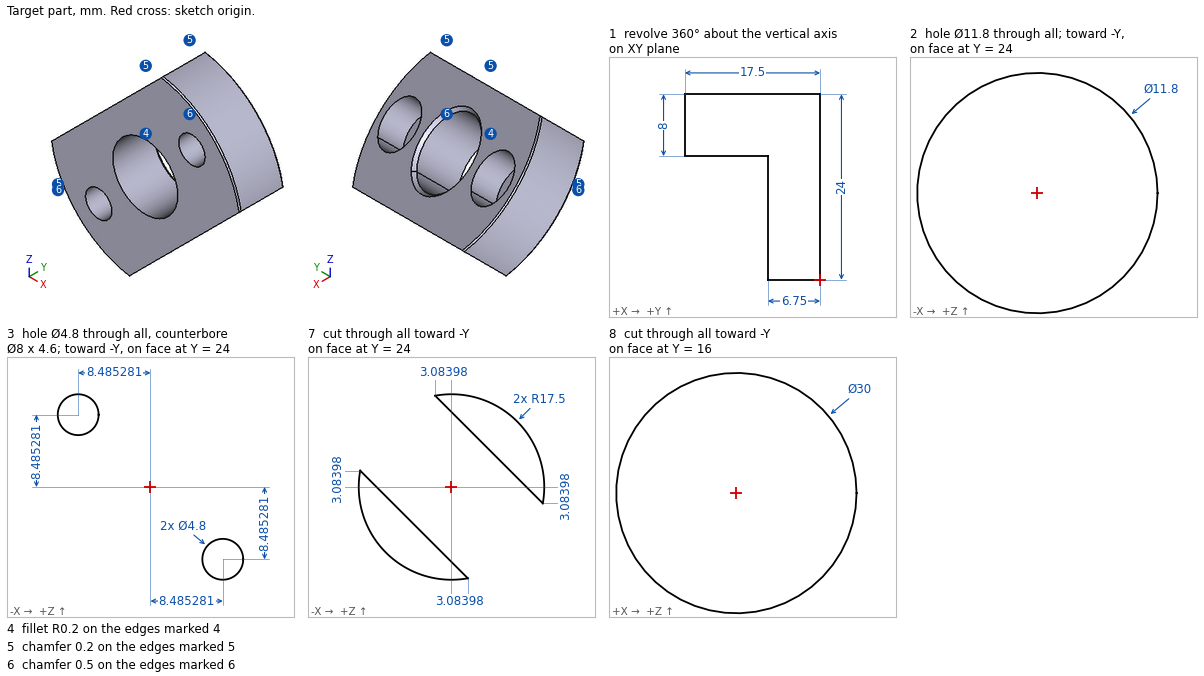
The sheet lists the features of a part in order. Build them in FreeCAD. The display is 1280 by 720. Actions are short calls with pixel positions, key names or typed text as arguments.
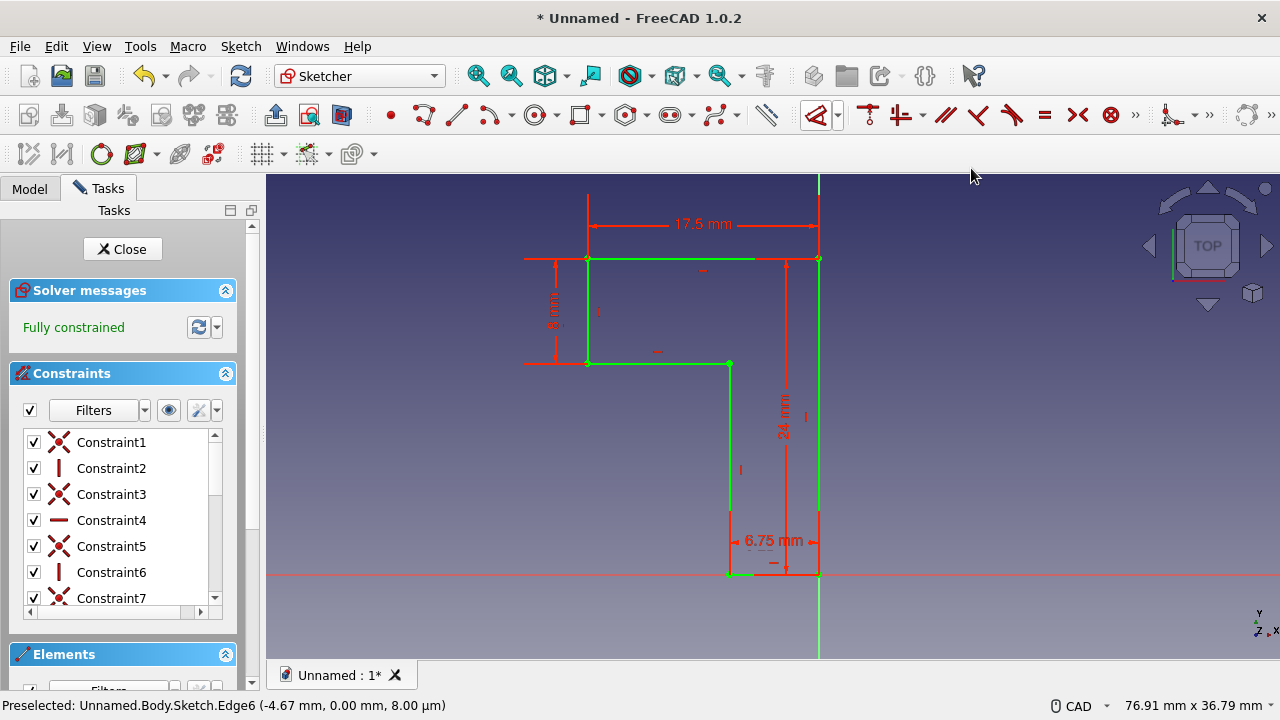
click(123, 249)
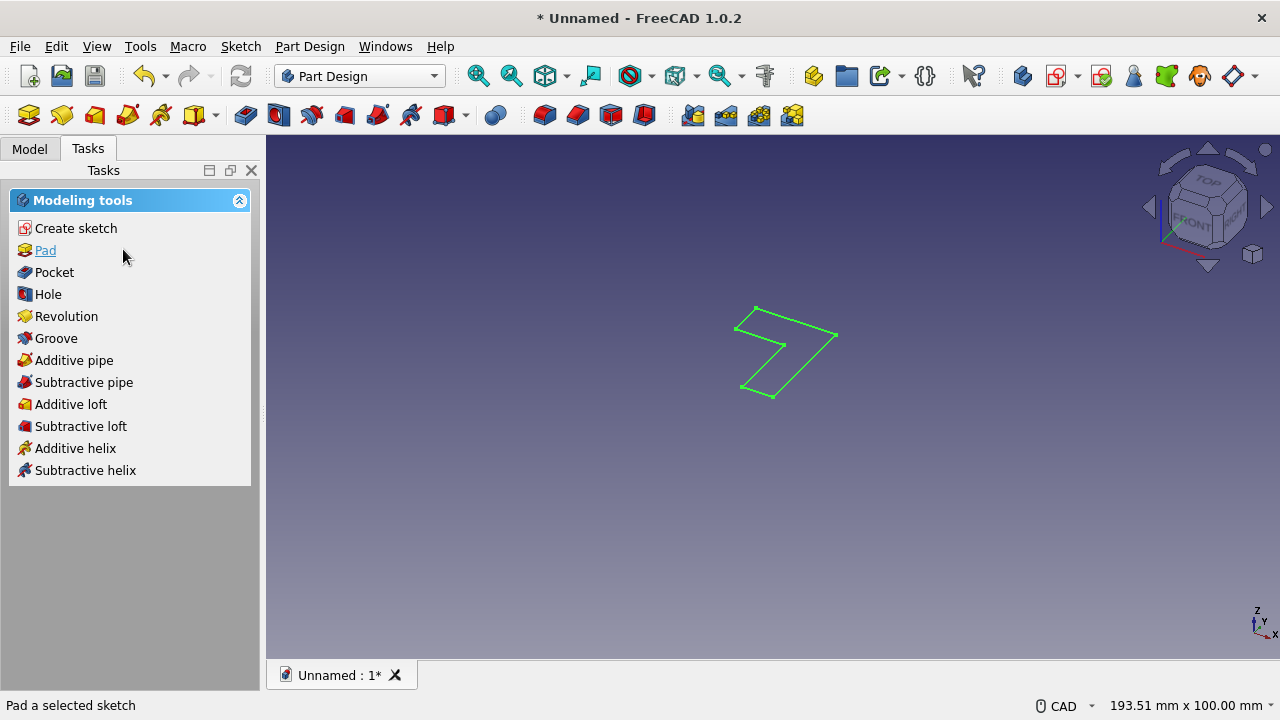
click(62, 116)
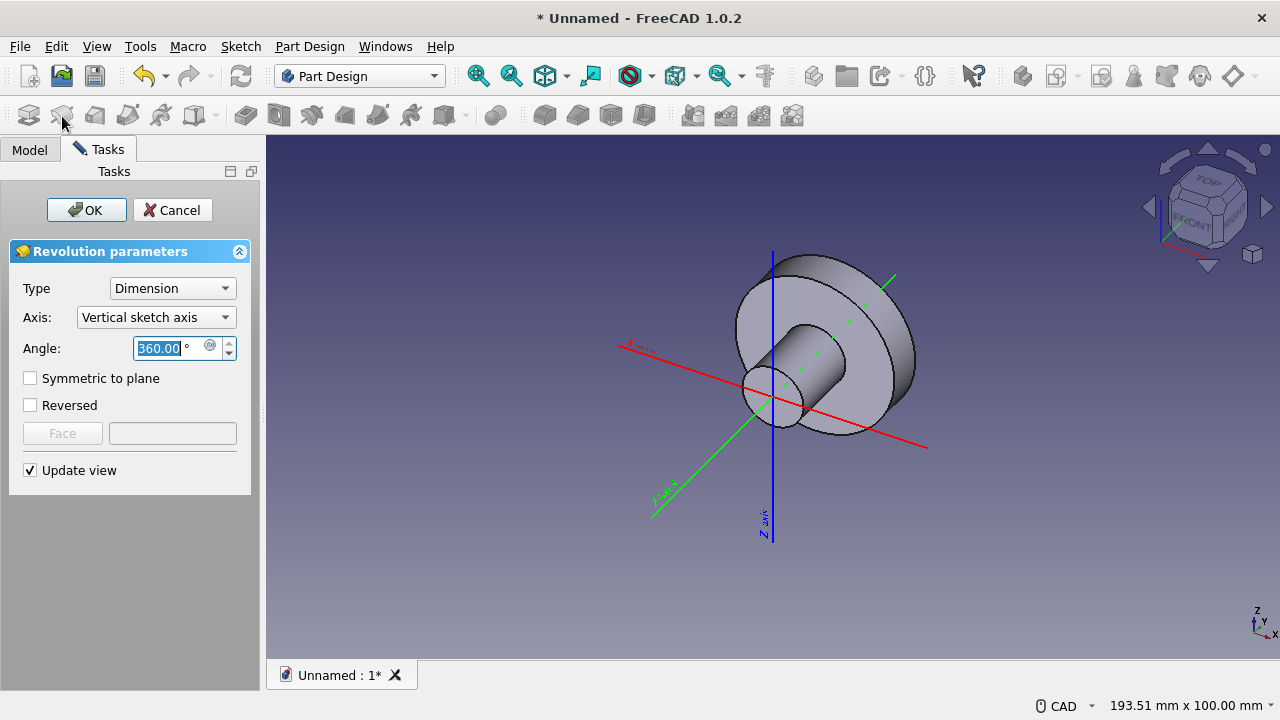
click(87, 210)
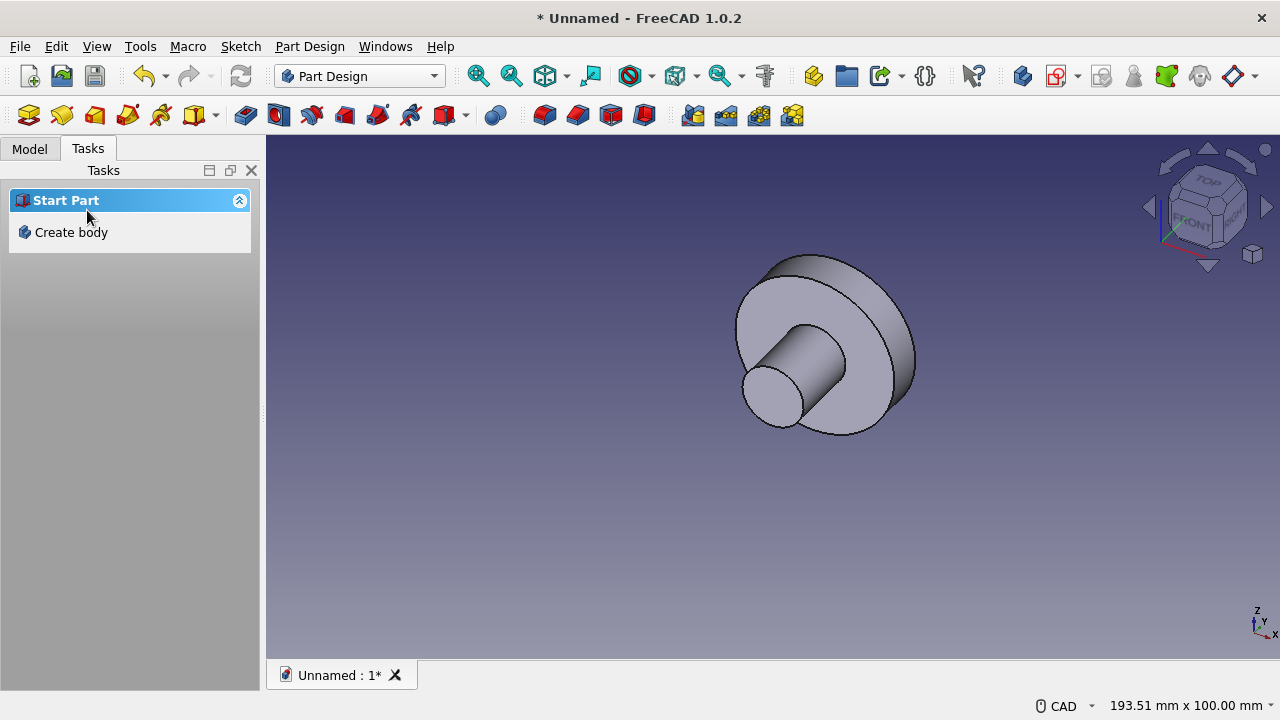
key(4)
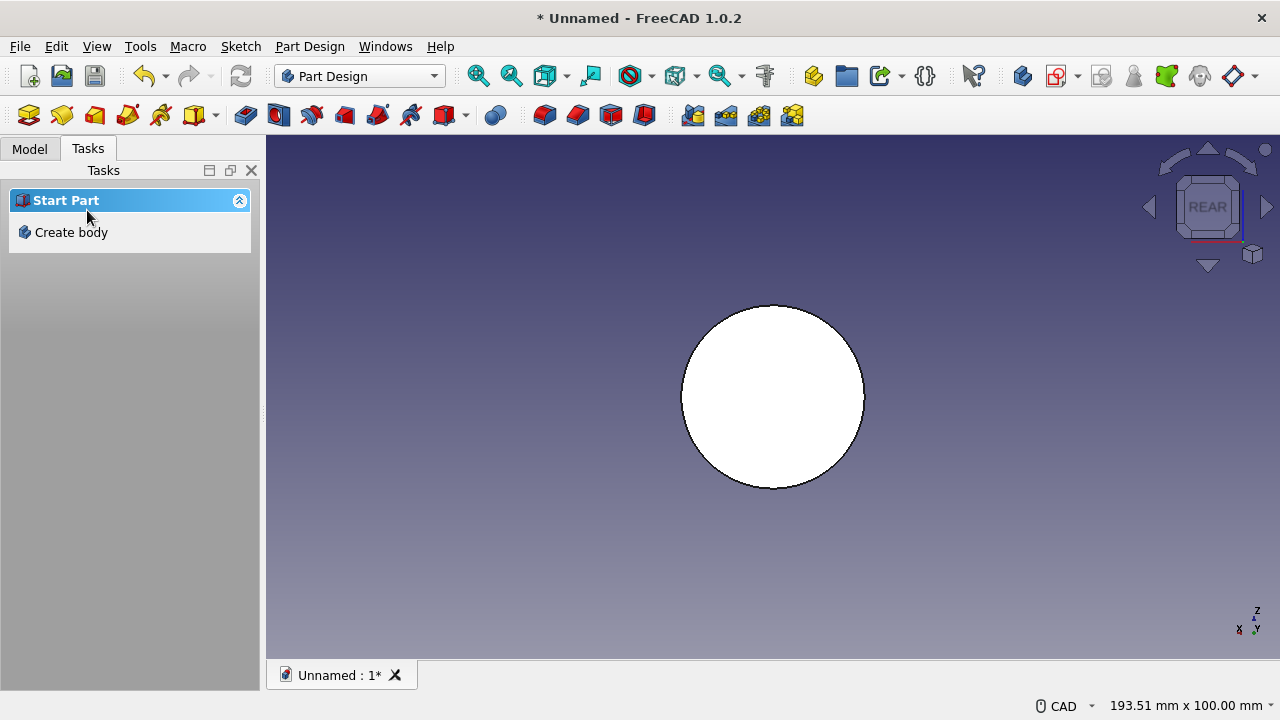
click(479, 76)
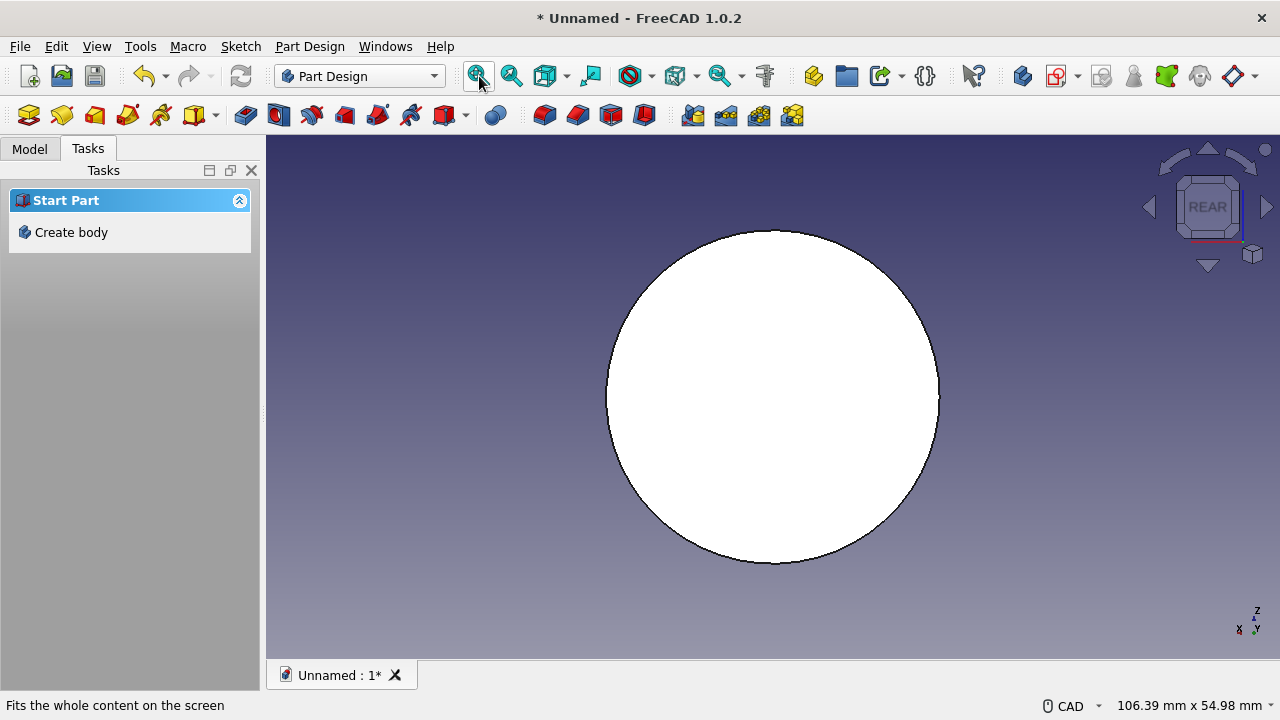
click(773, 396)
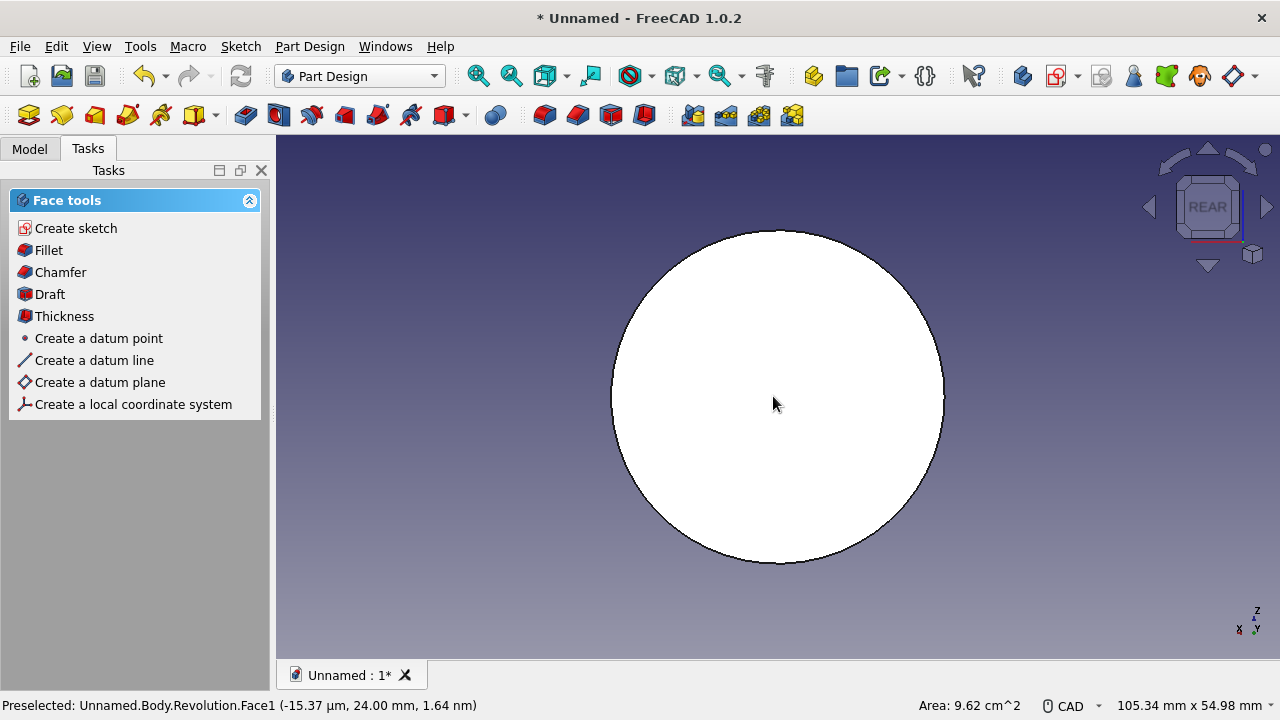
click(1056, 76)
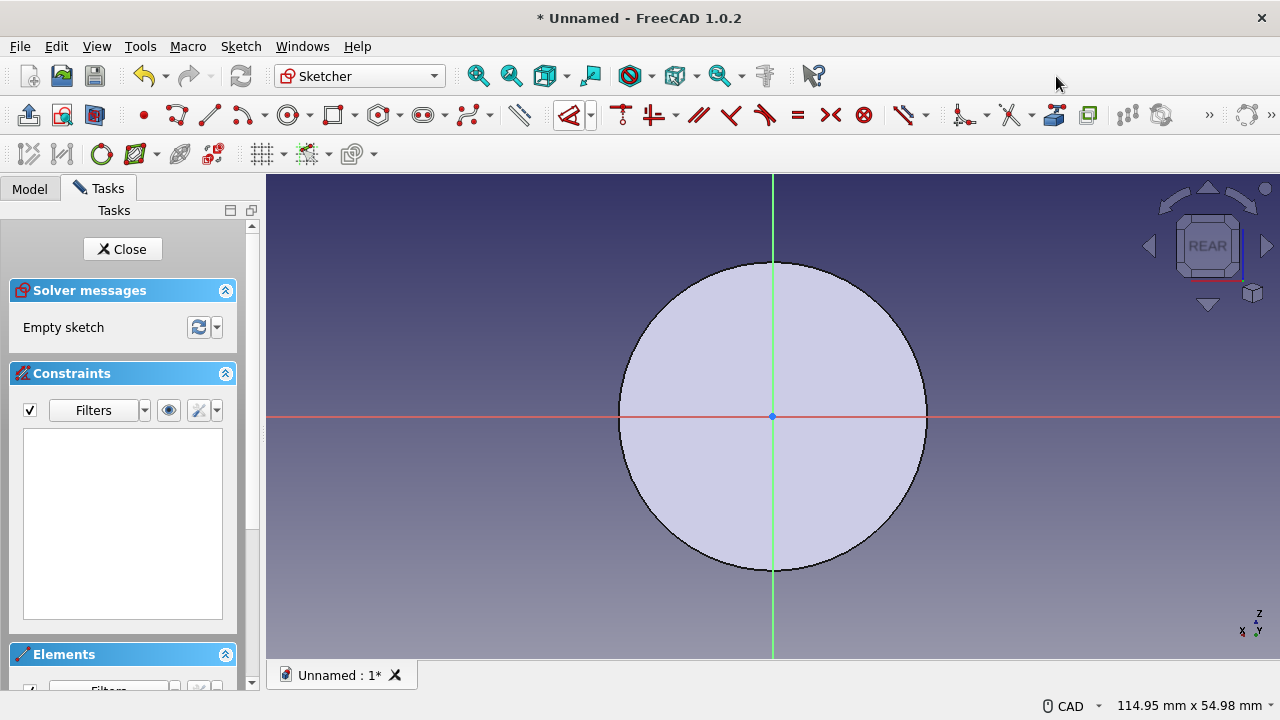
scroll(813, 416, up, 5)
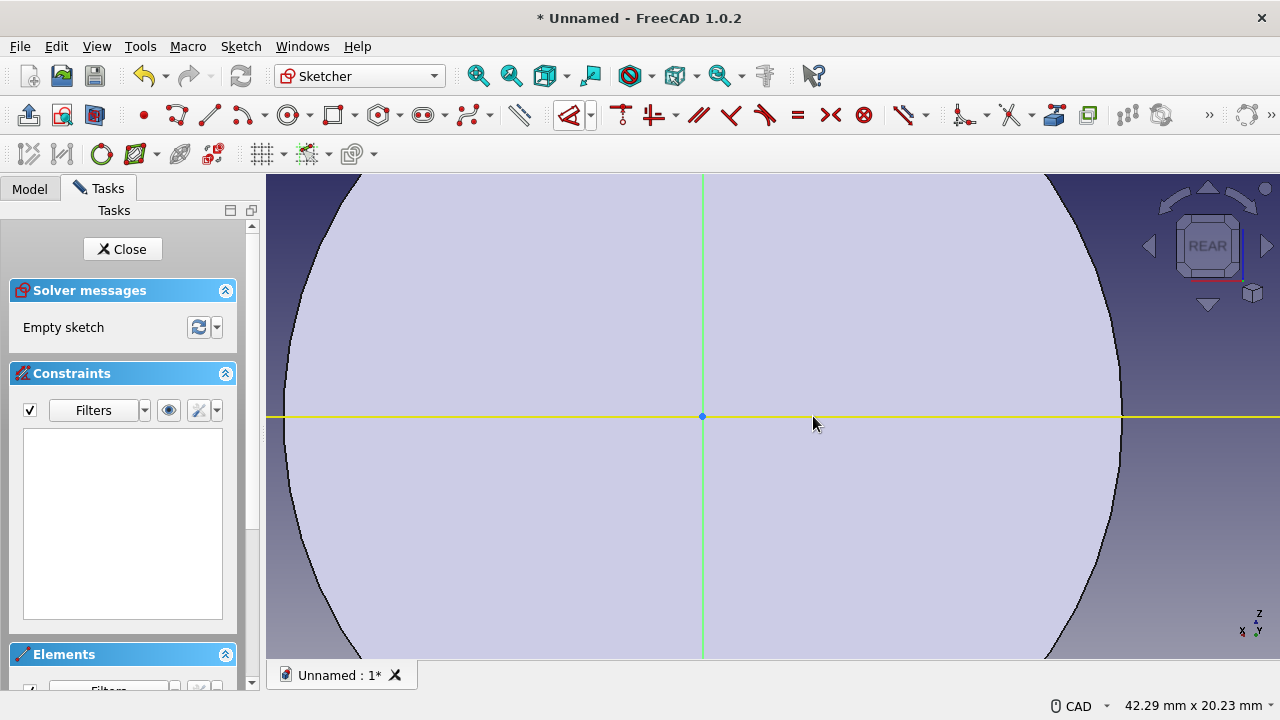
key(g)
key(c)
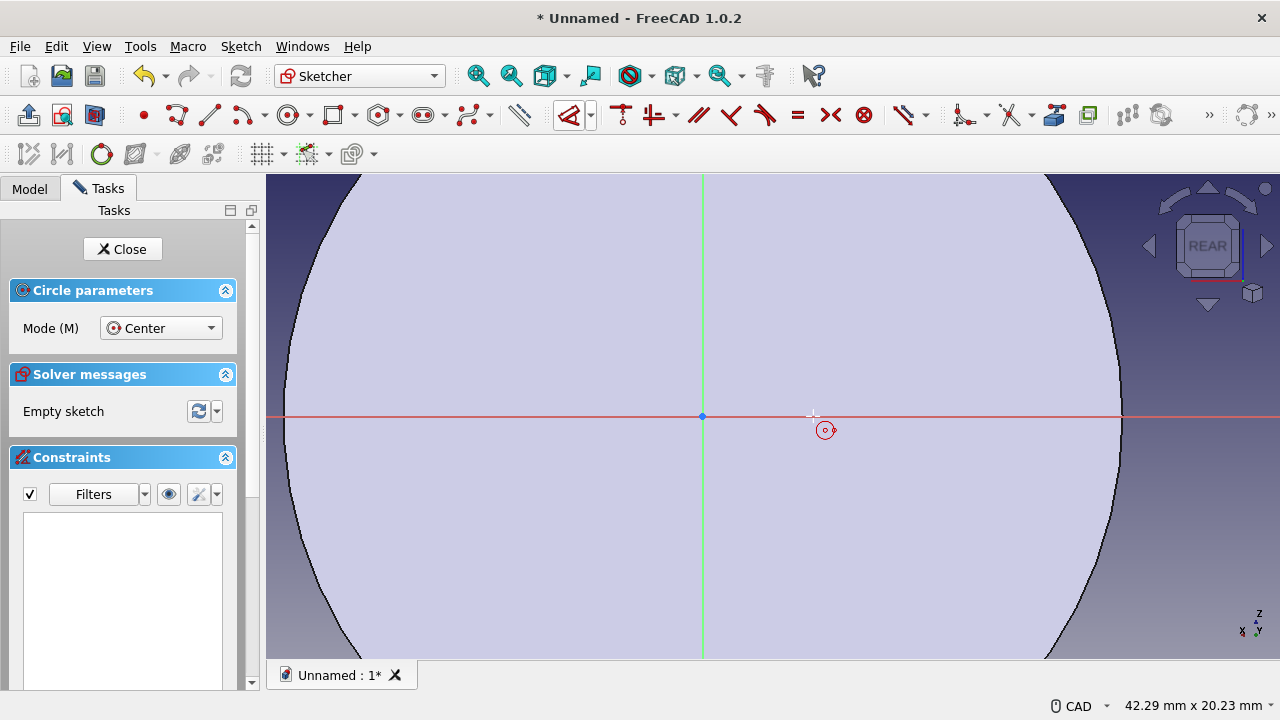
click(703, 416)
move(803, 316)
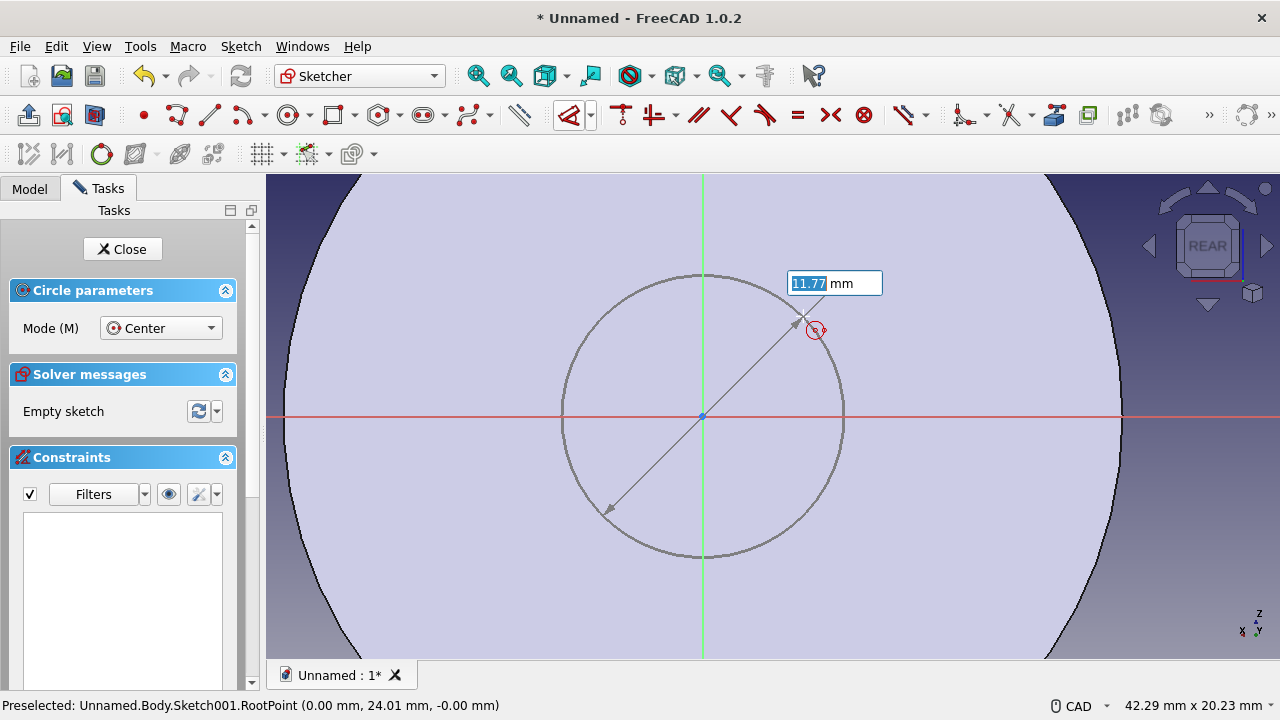
text(11.8)
key(Return)
key(Escape)